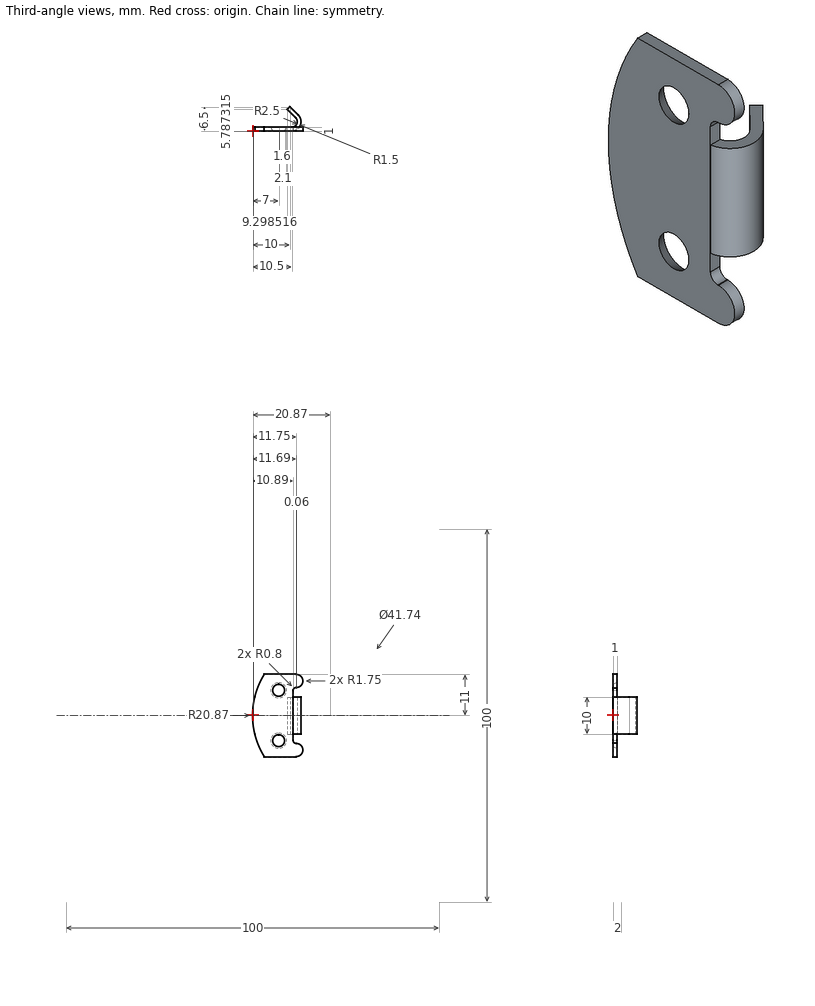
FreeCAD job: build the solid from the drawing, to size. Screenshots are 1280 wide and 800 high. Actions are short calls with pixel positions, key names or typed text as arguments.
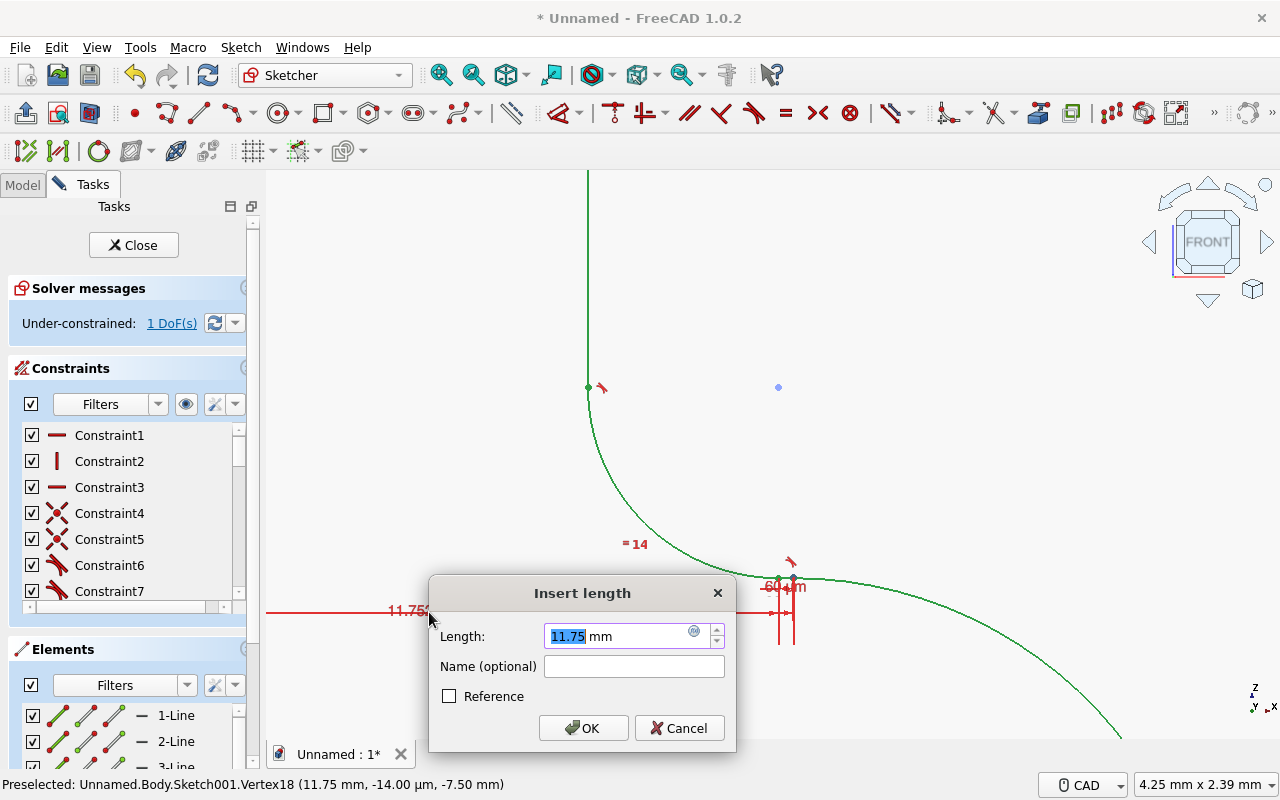
text(11.69)
key(Return)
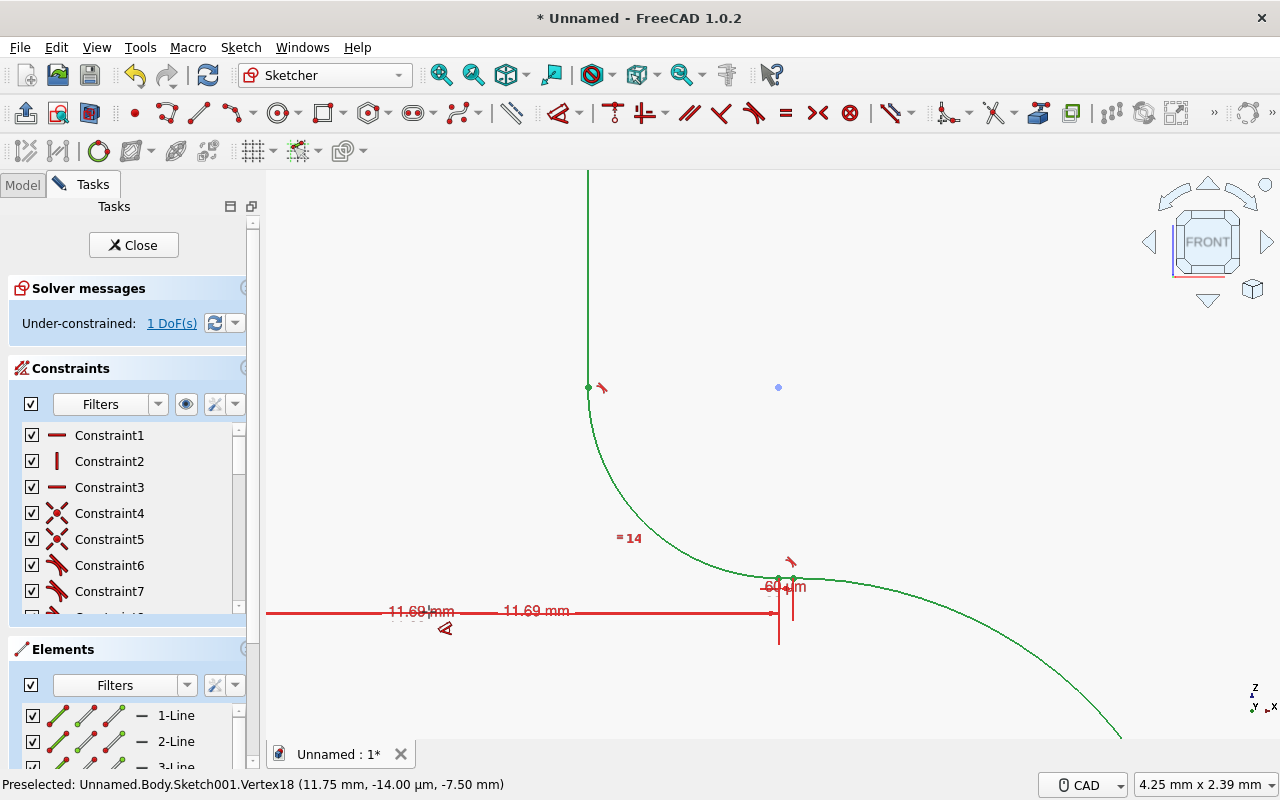
scroll(793, 588, down, 13)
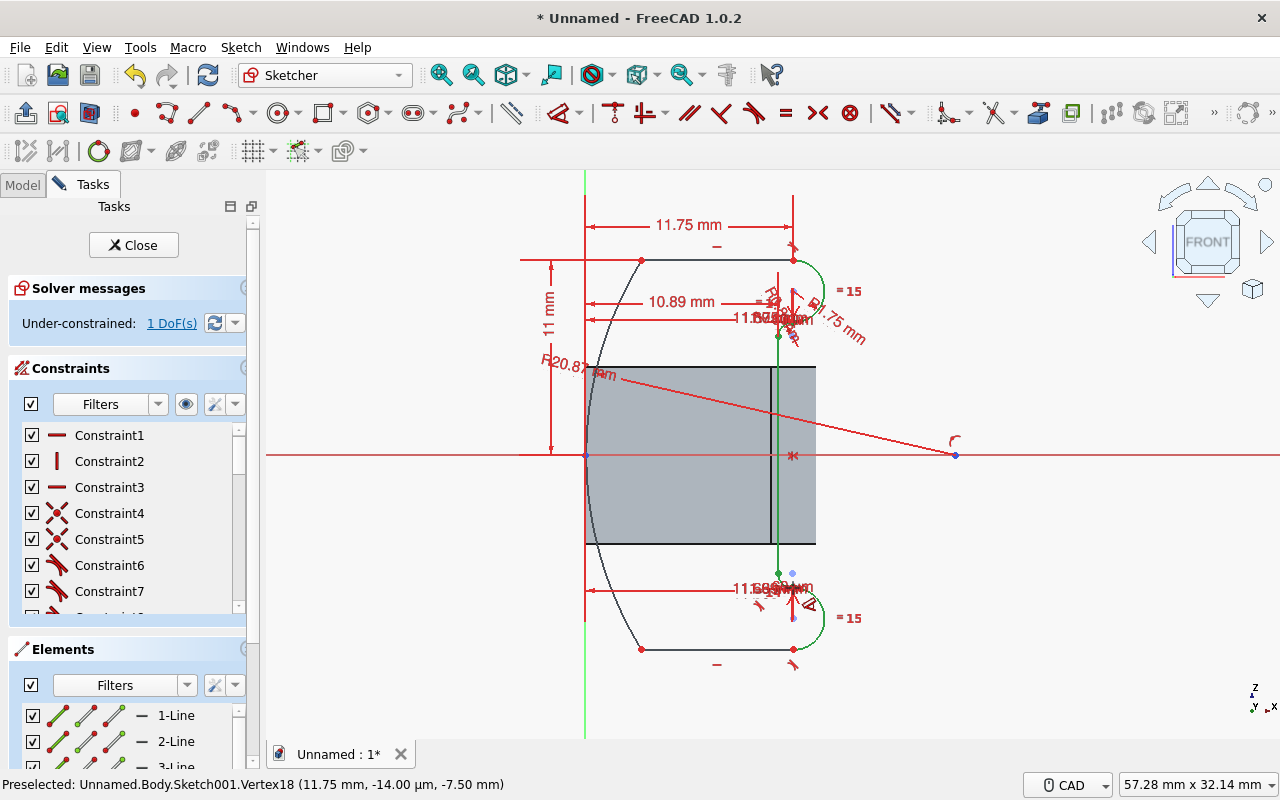
click(956, 455)
click(685, 489)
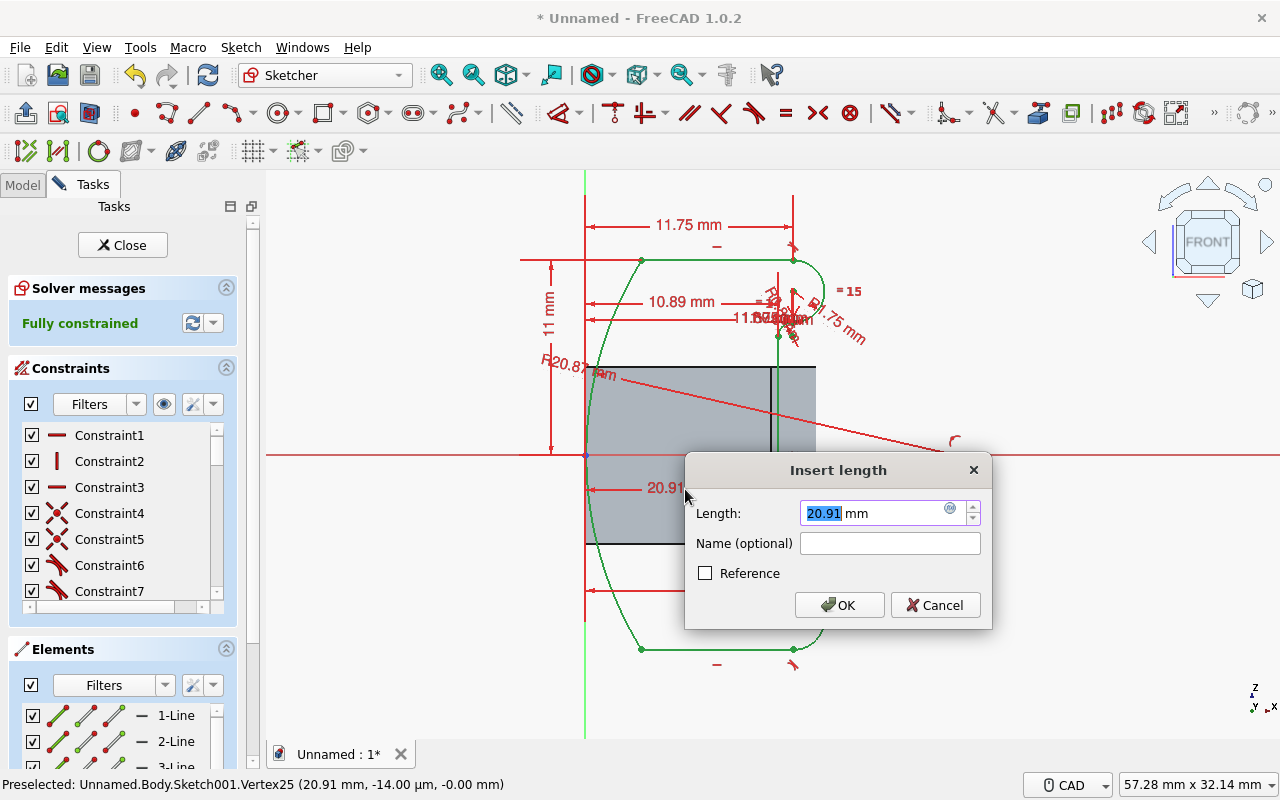
text(20.87)
key(Return)
key(Escape)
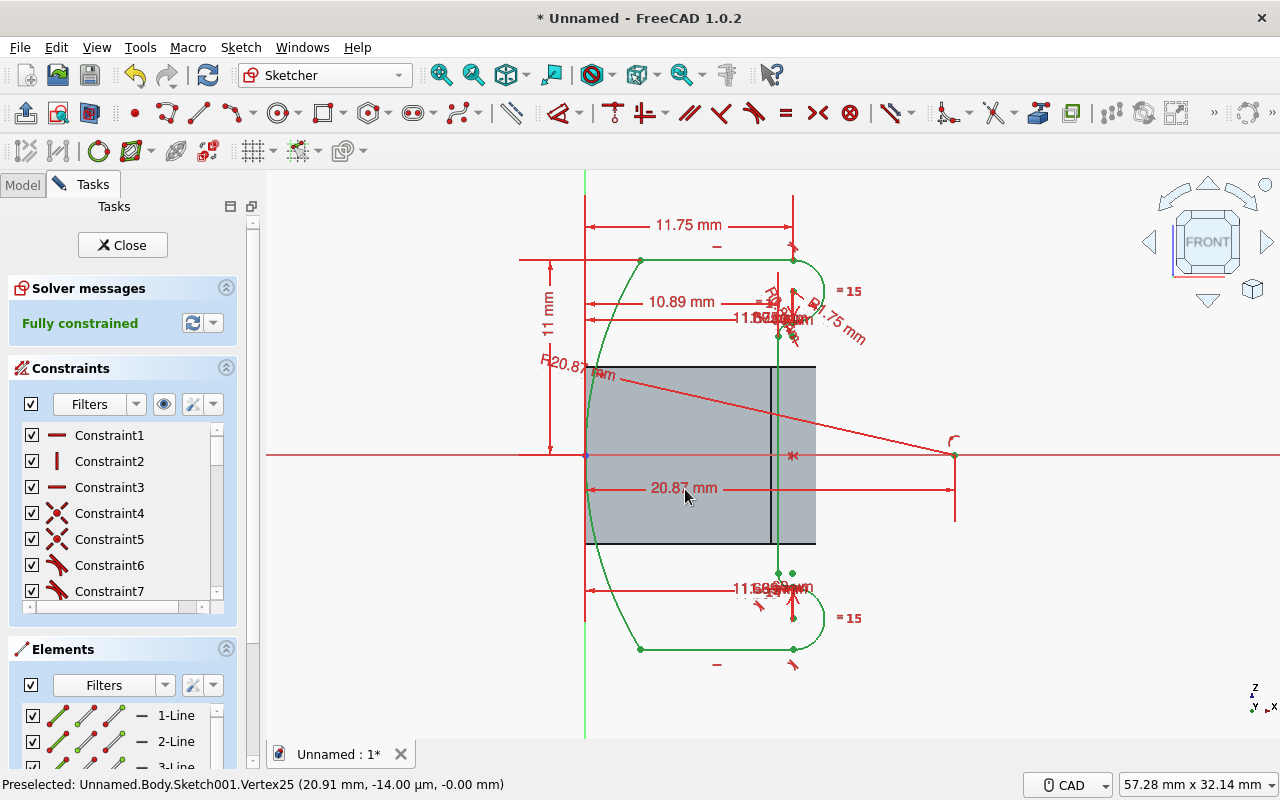
click(123, 245)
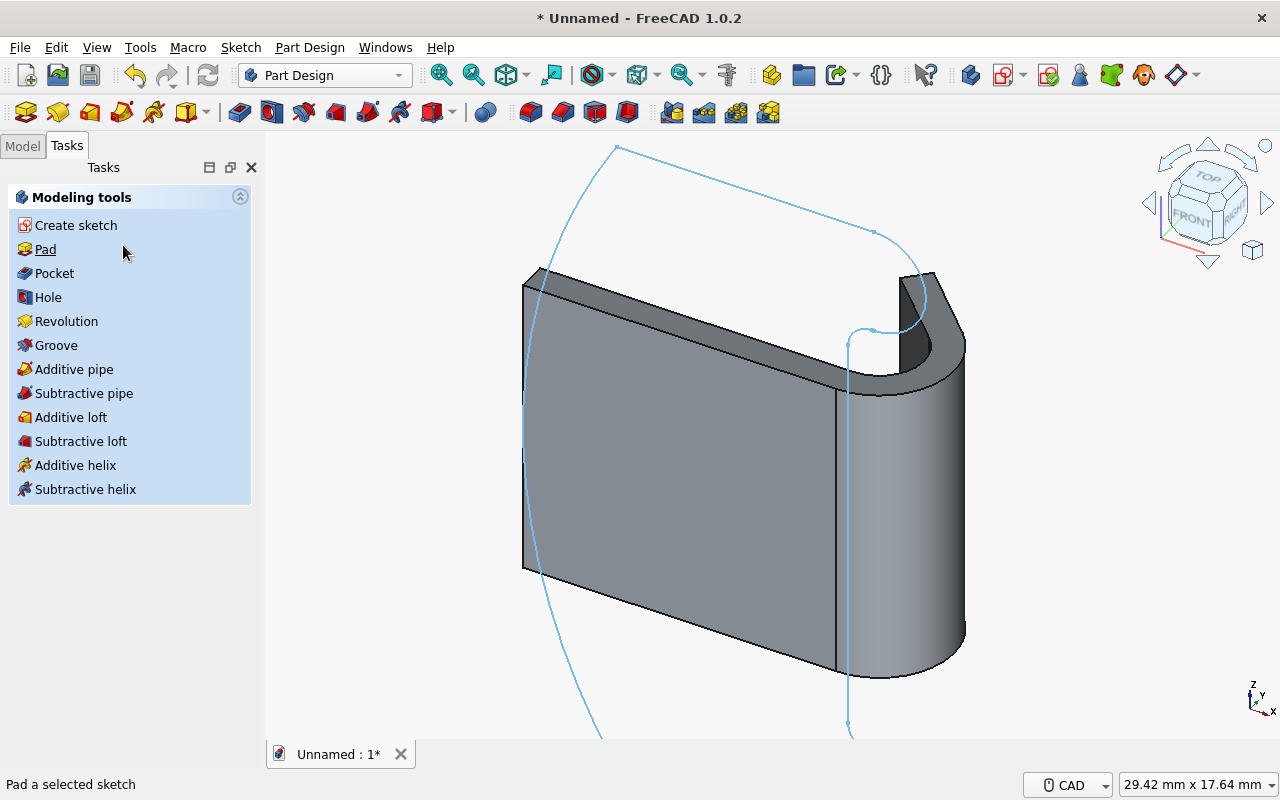
click(26, 112)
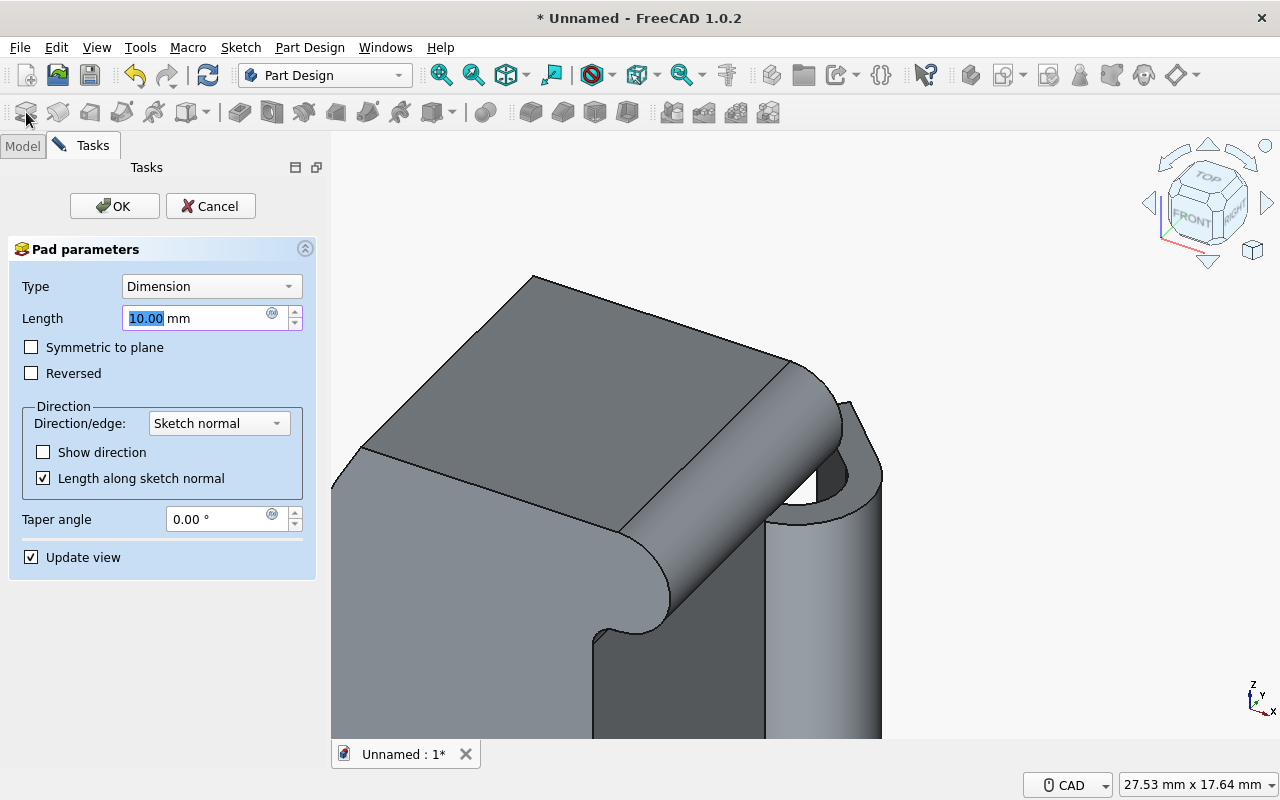
text(1)
key(Tab)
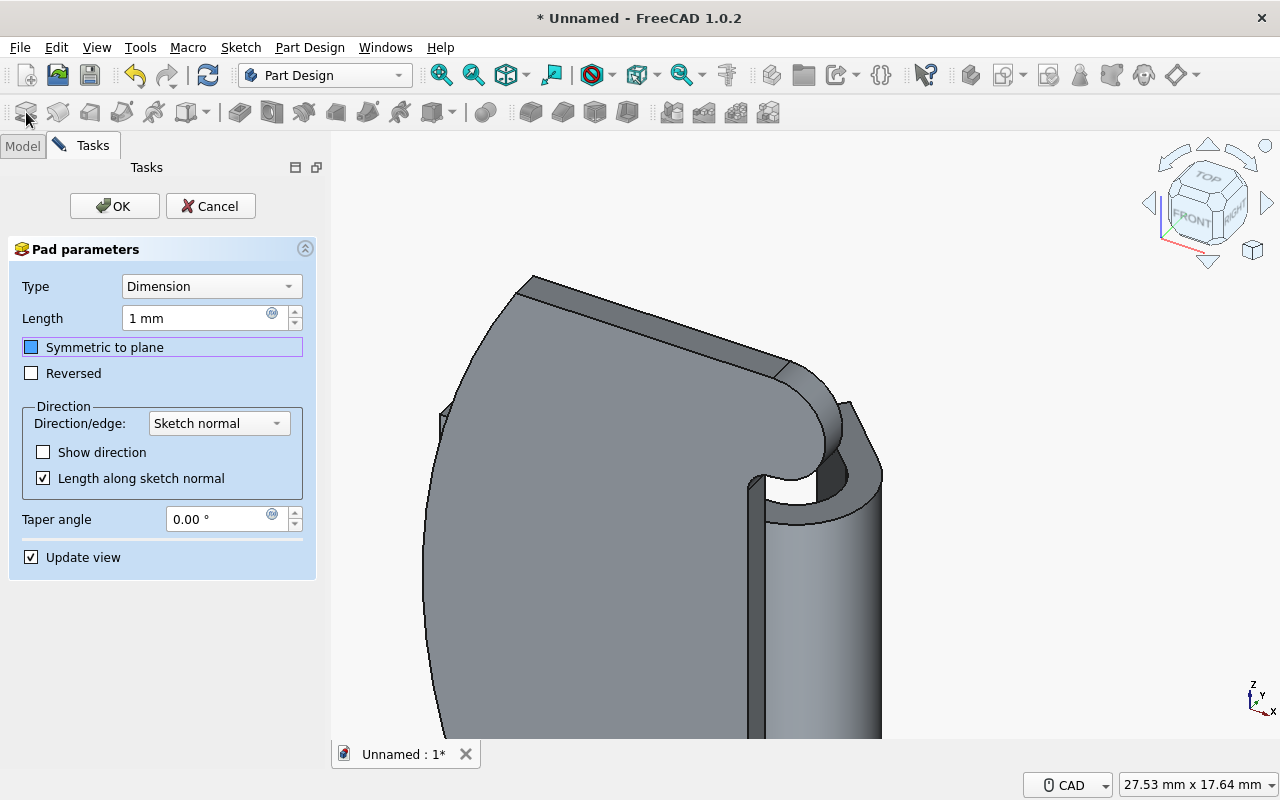
click(30, 373)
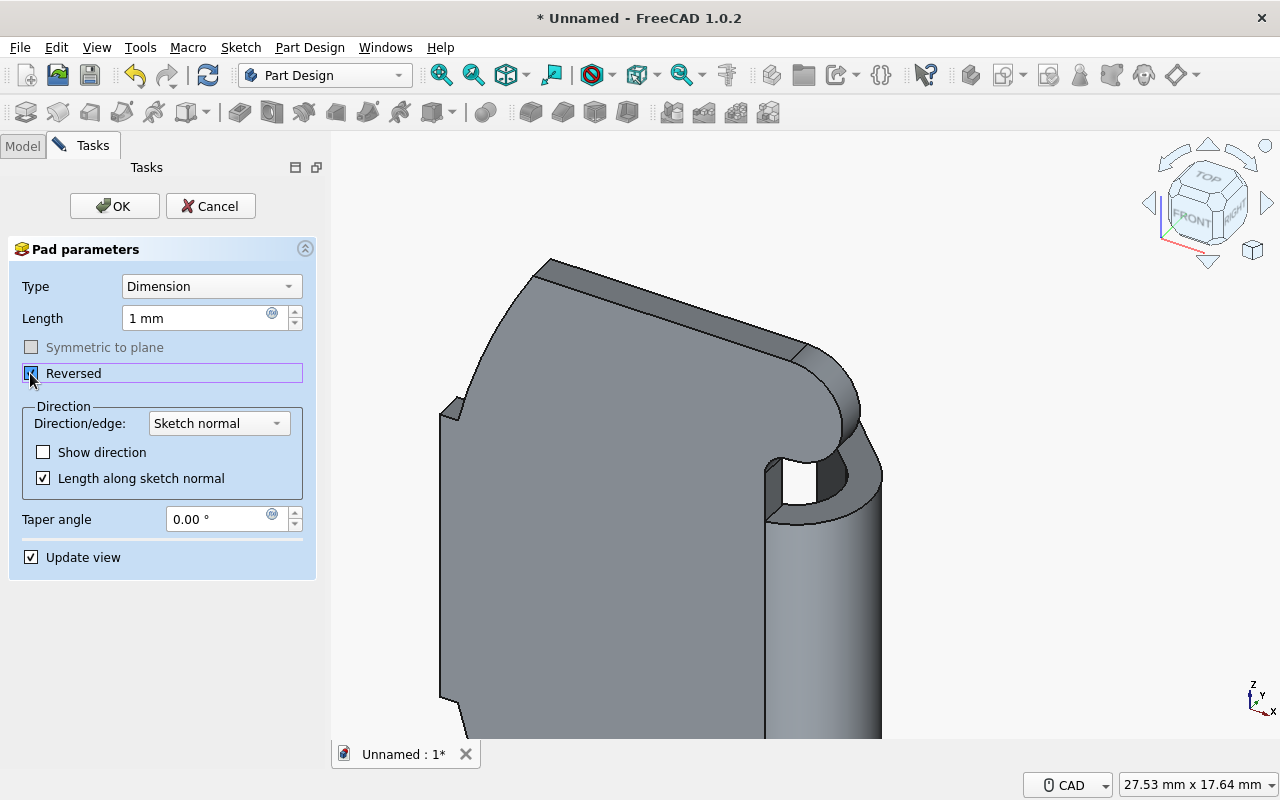
click(115, 206)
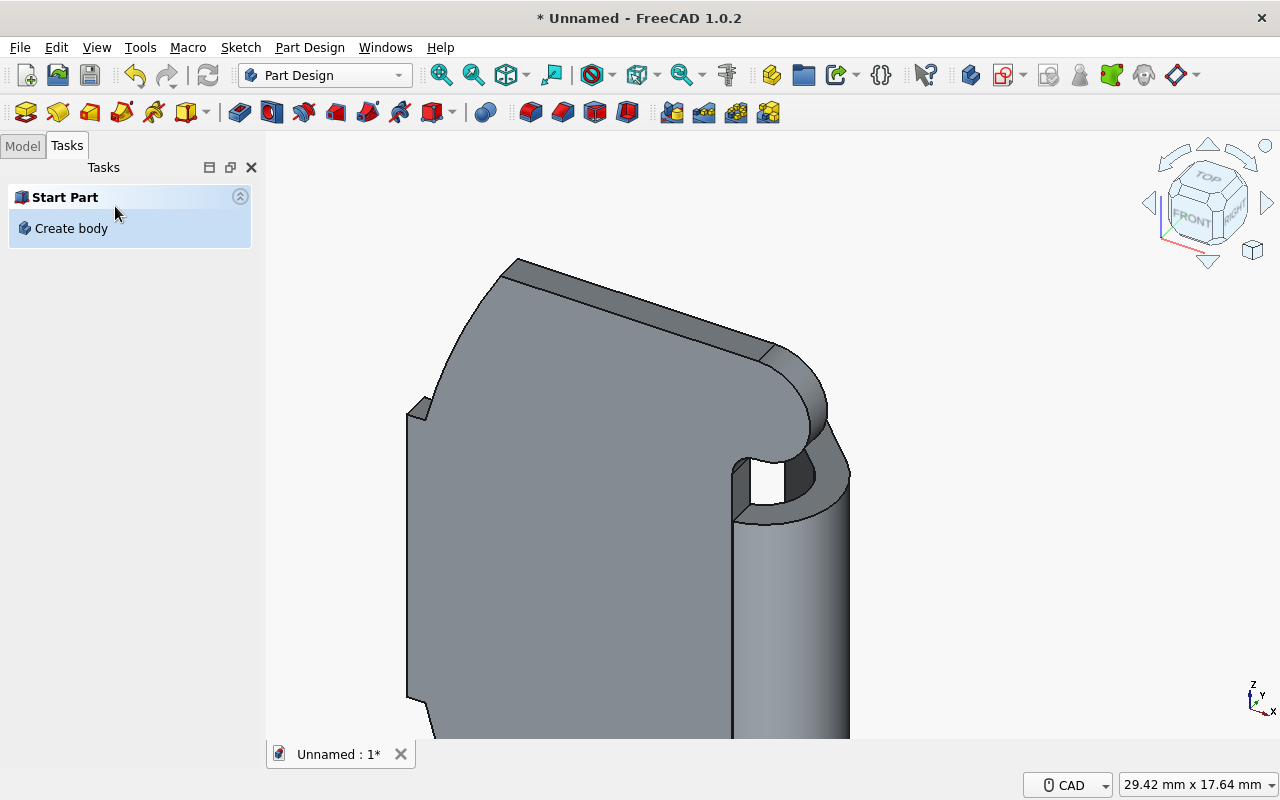
click(442, 76)